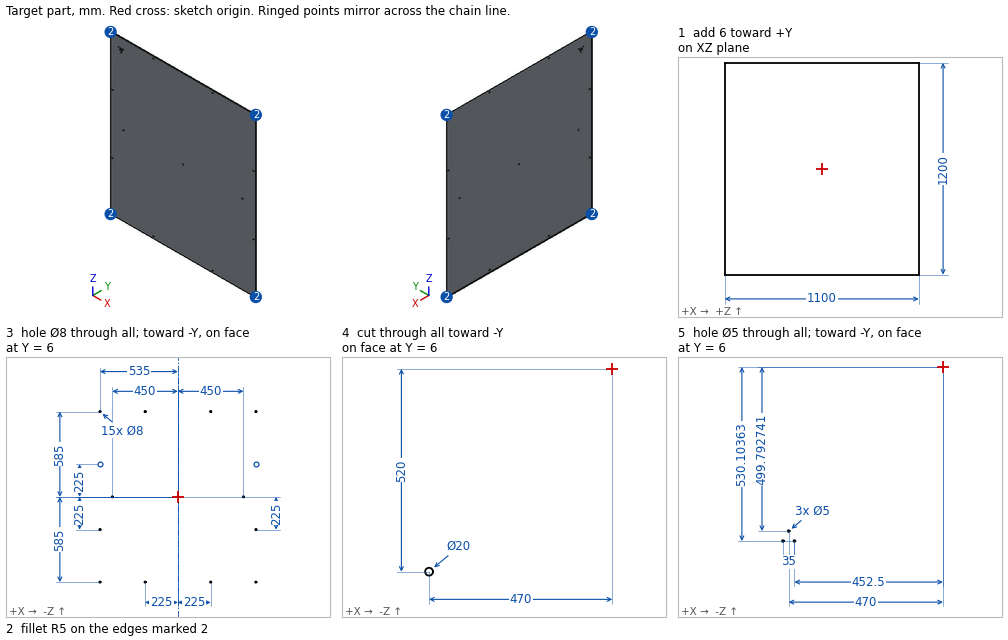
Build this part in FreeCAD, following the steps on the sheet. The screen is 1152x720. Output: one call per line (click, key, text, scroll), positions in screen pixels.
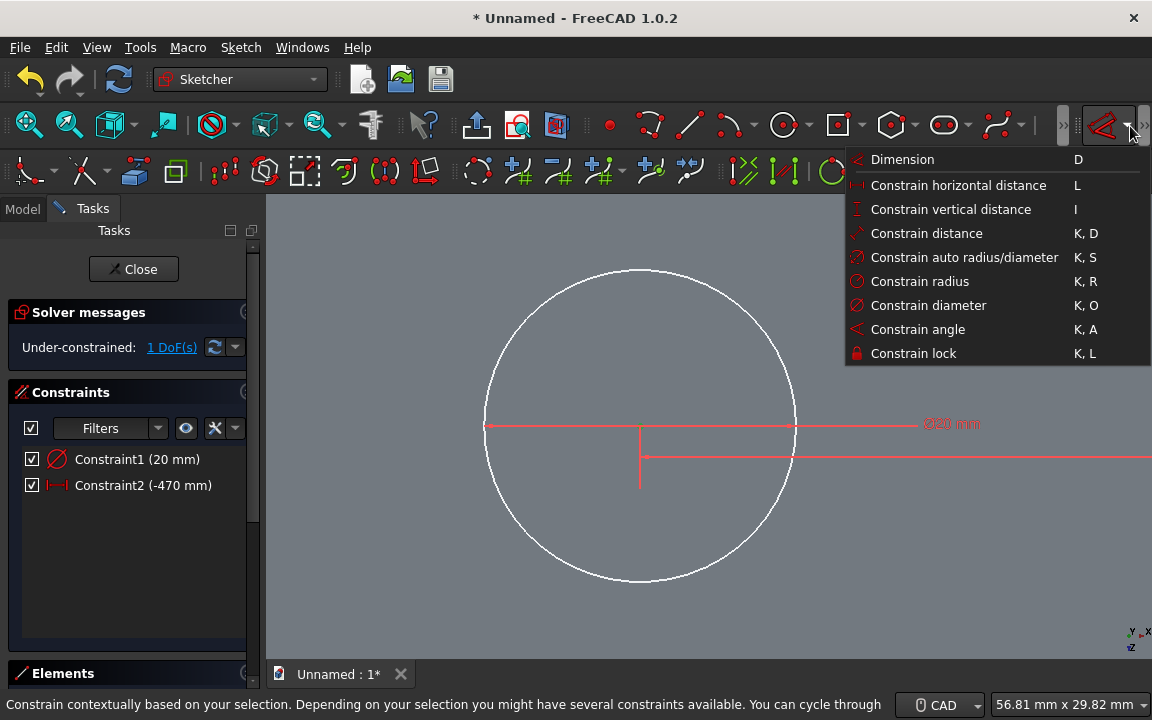
click(998, 209)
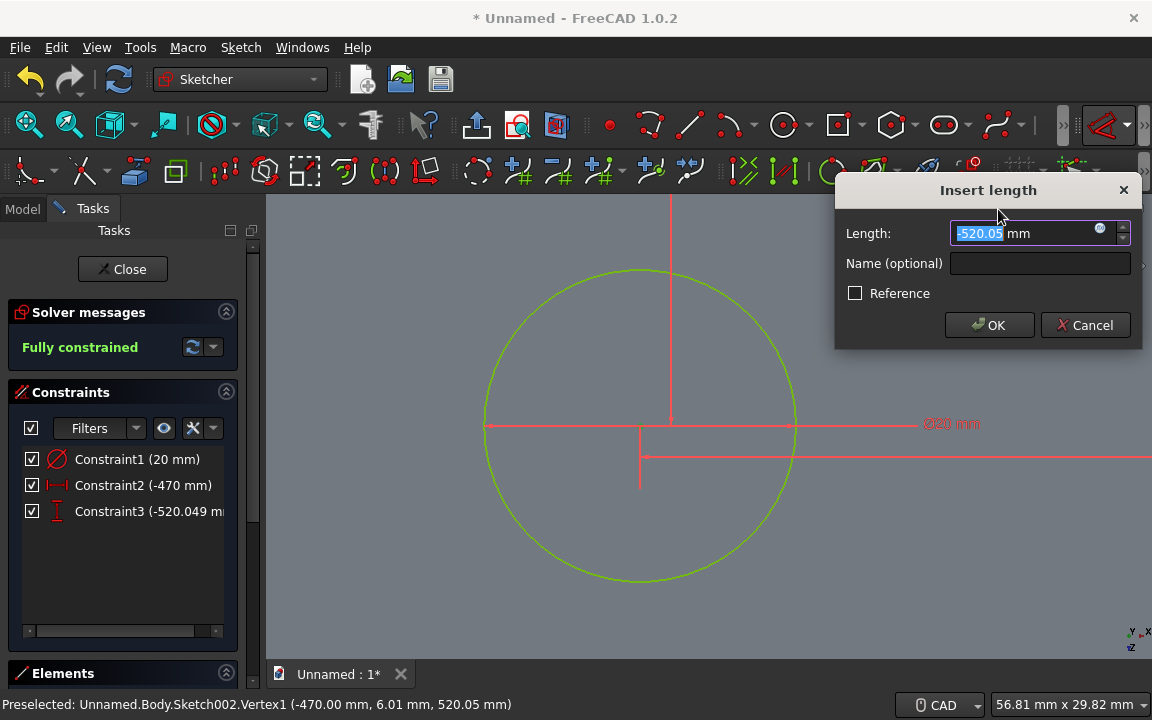
text(-520)
key(Return)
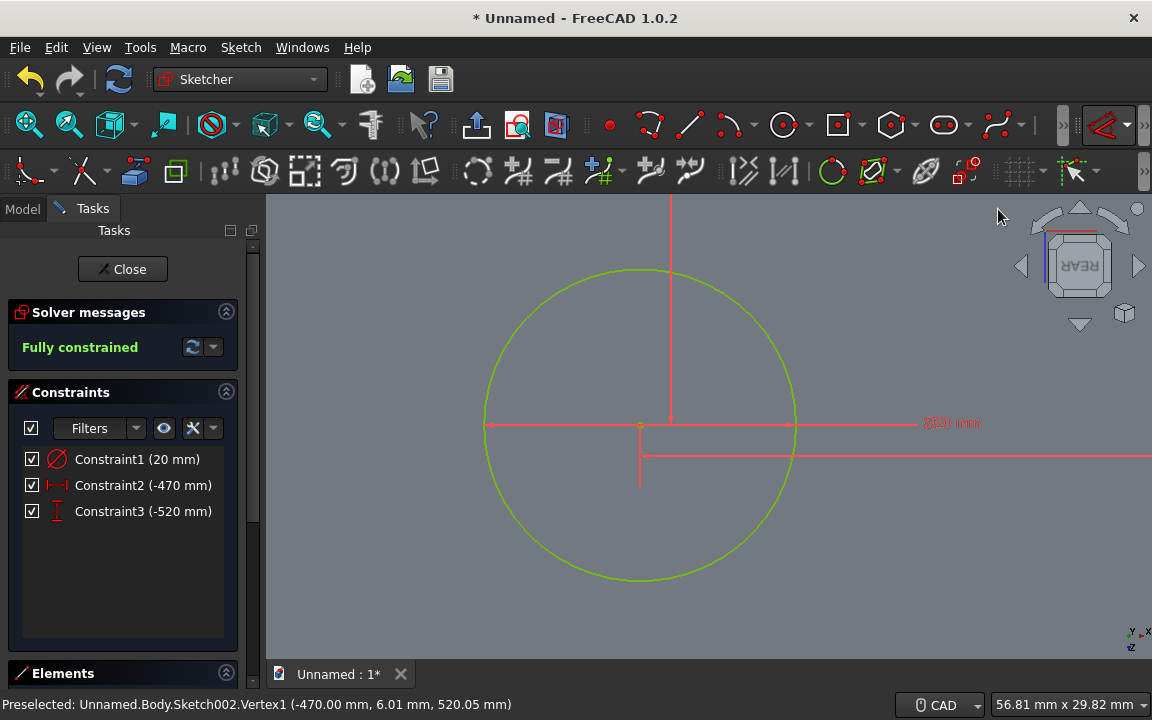
click(123, 269)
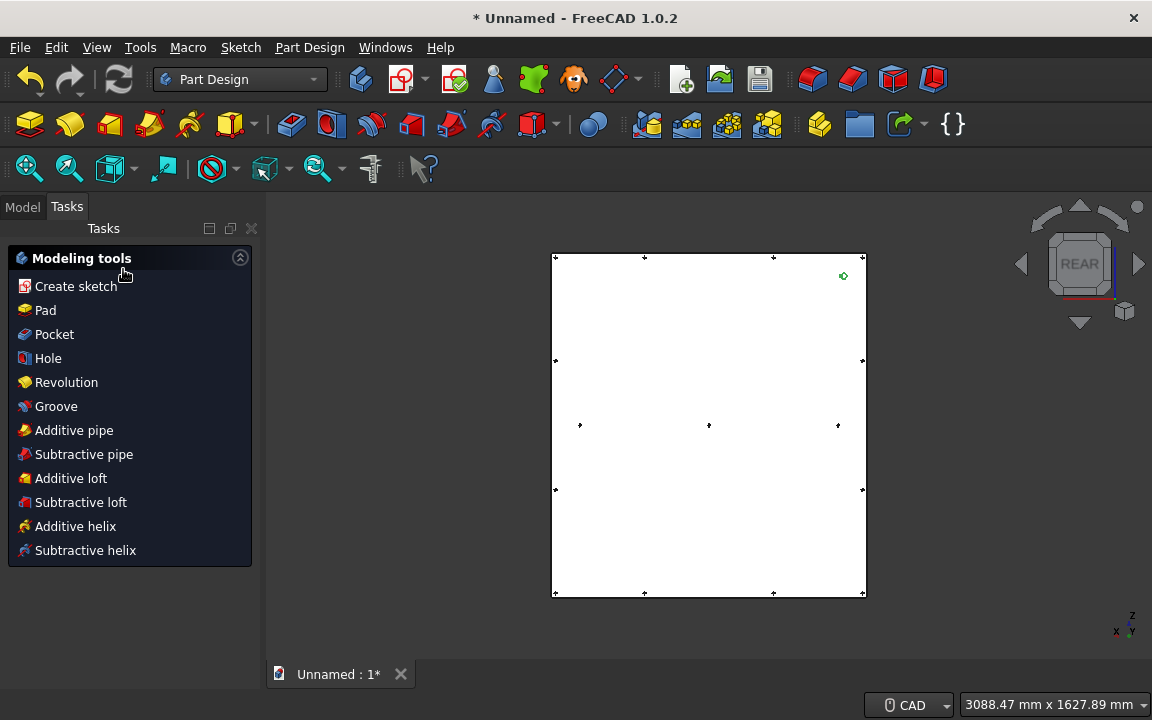
click(292, 124)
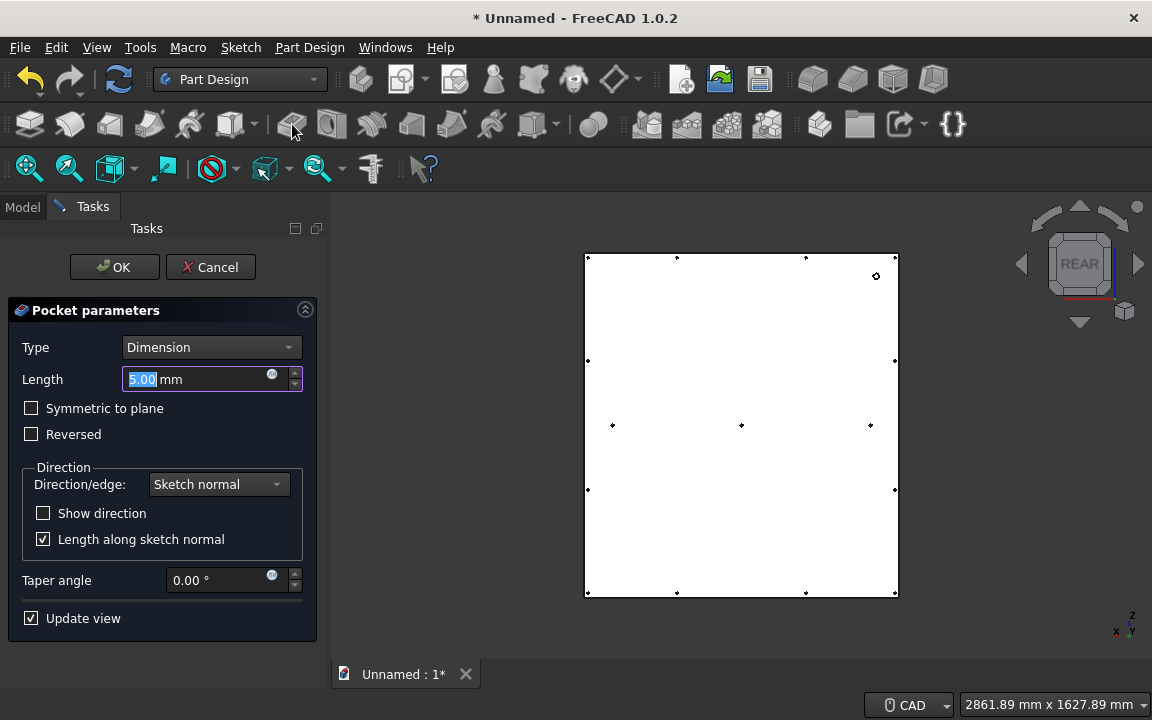
click(212, 348)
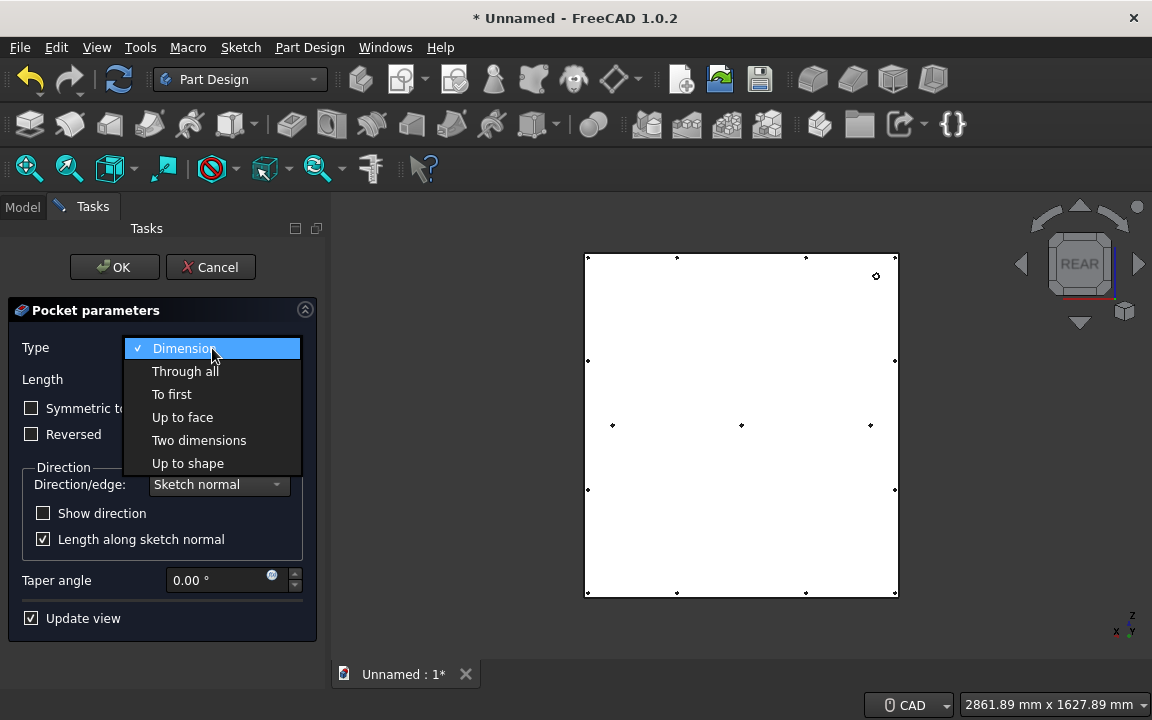
click(212, 372)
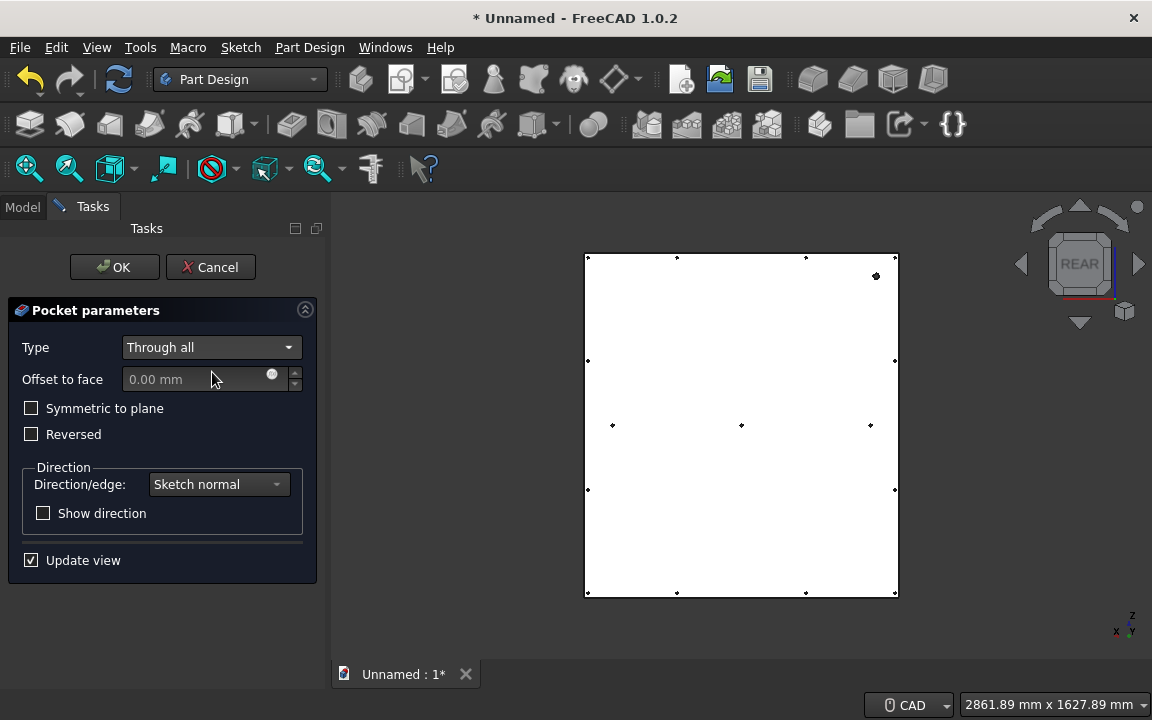
click(115, 267)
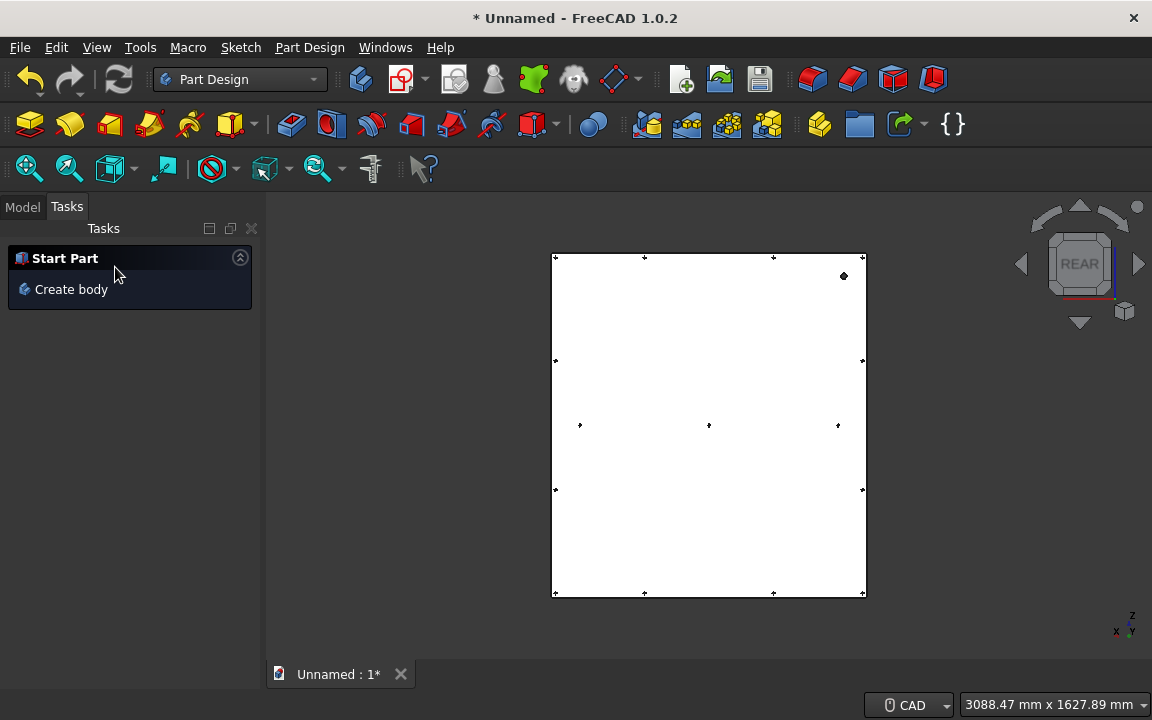
click(709, 523)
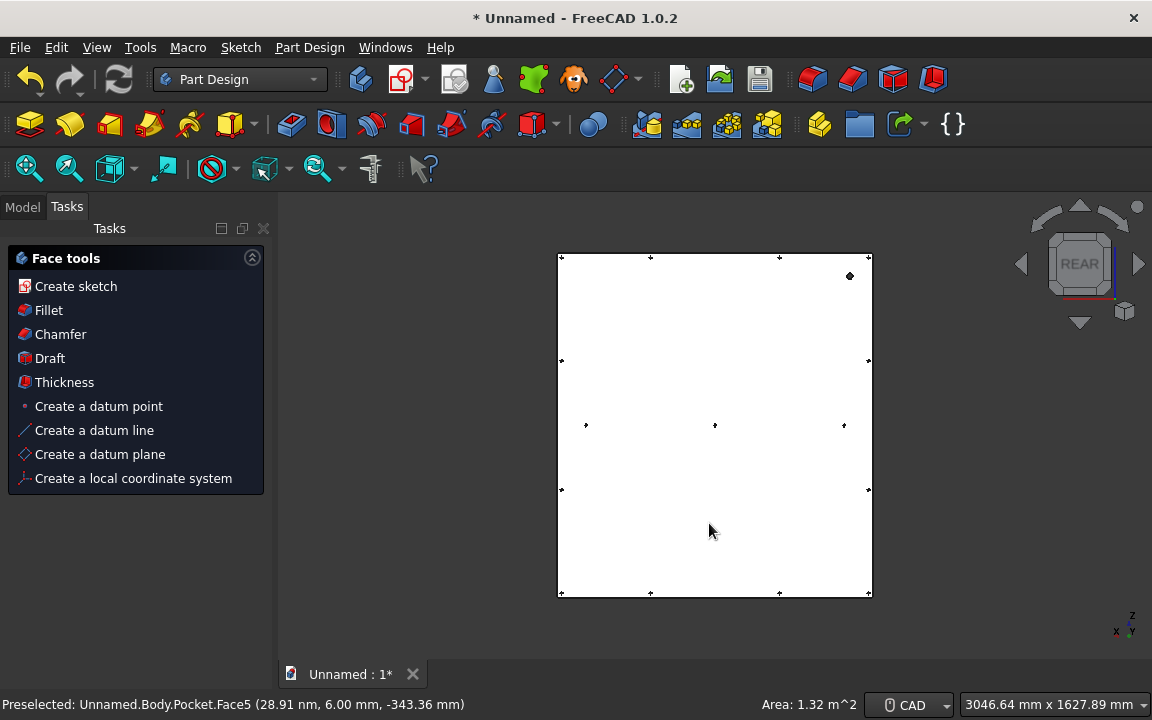
click(402, 80)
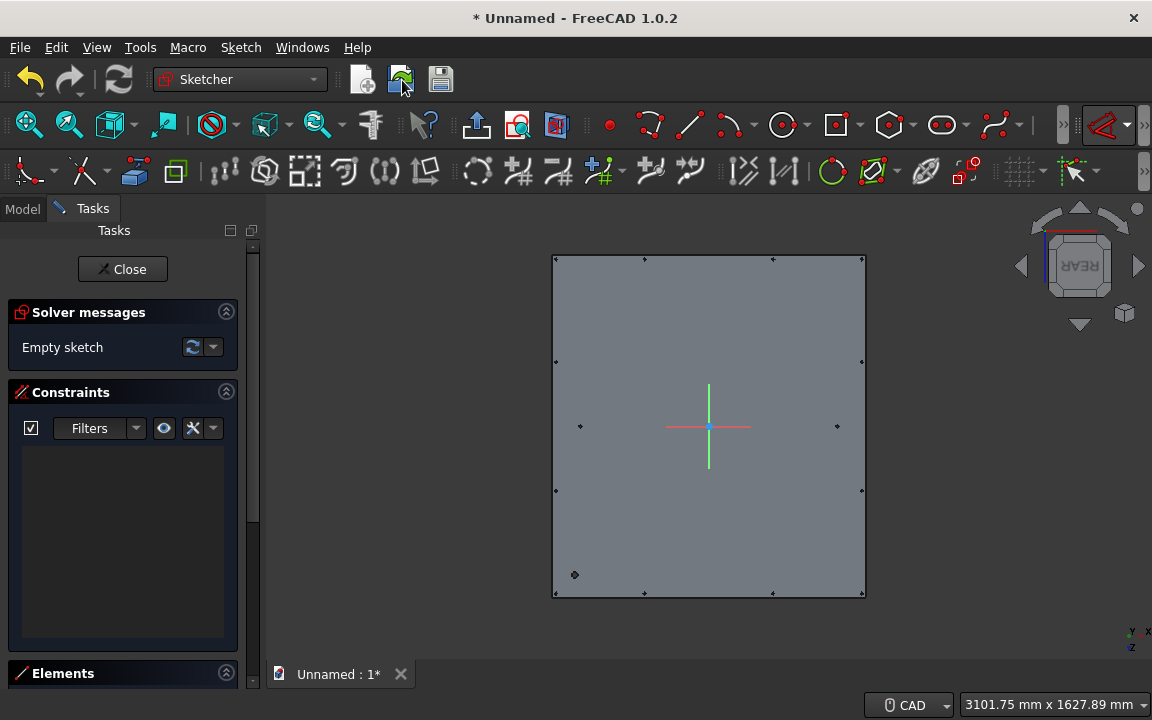
scroll(571, 581, up, 15)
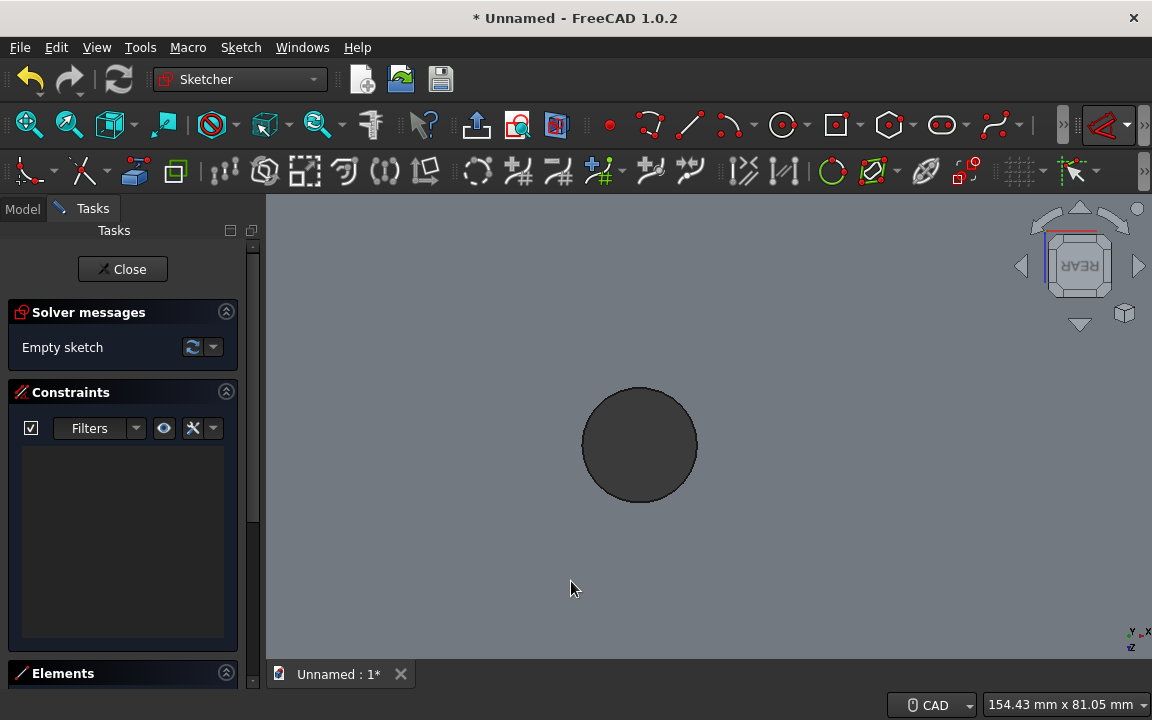
scroll(638, 396, up, 2)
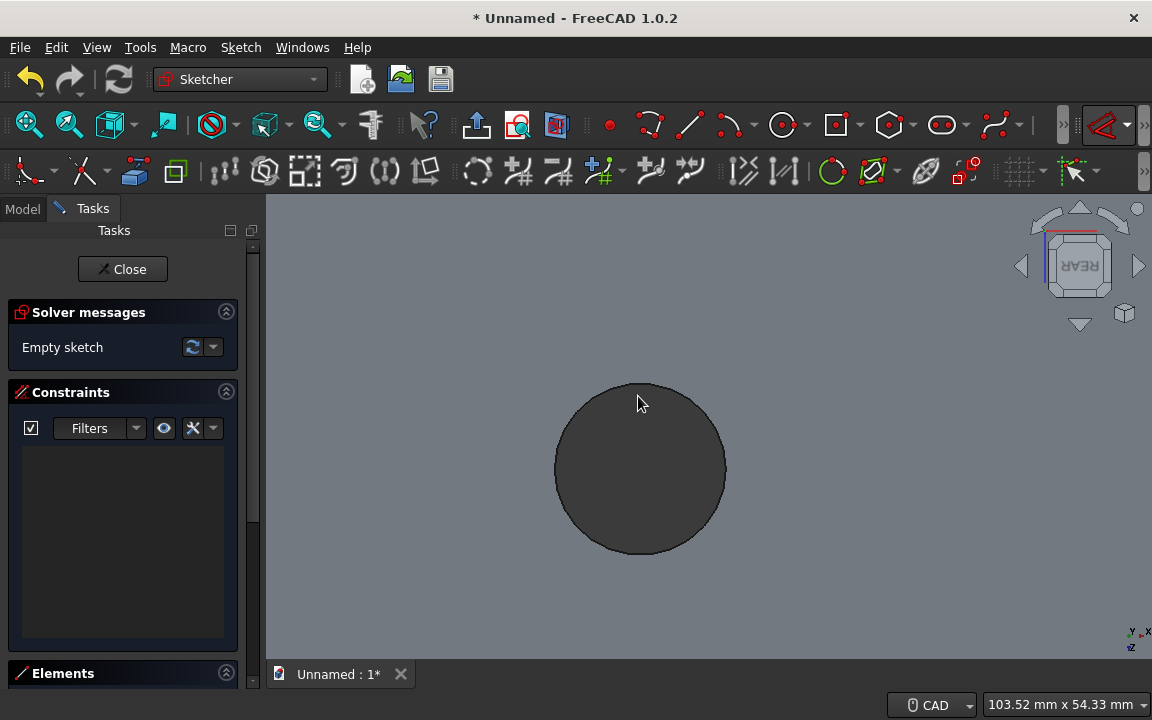
click(784, 126)